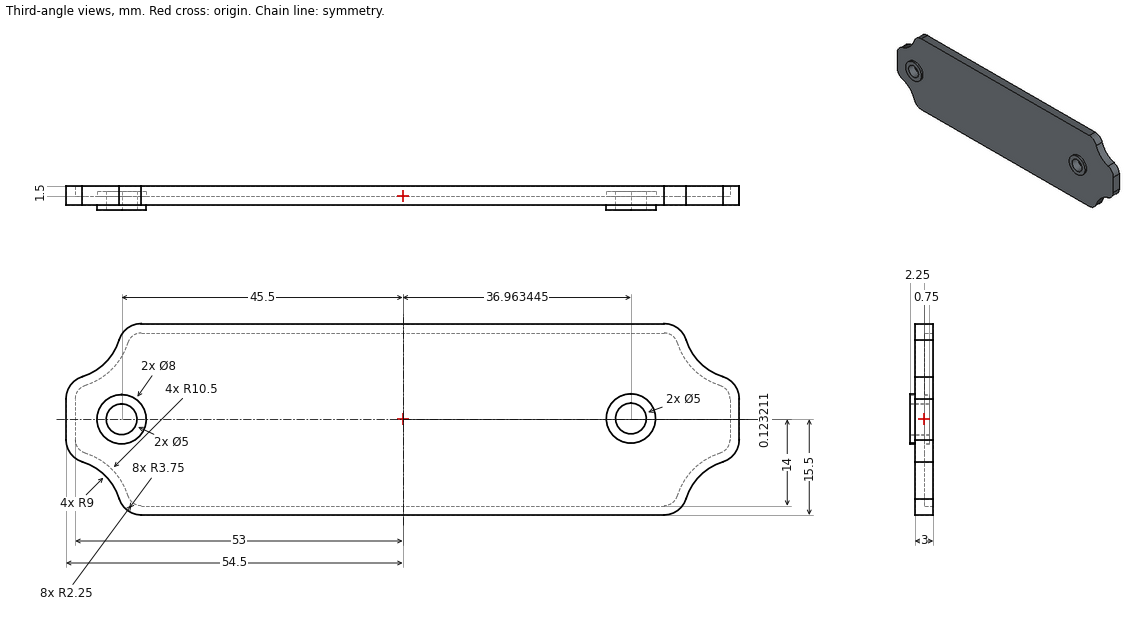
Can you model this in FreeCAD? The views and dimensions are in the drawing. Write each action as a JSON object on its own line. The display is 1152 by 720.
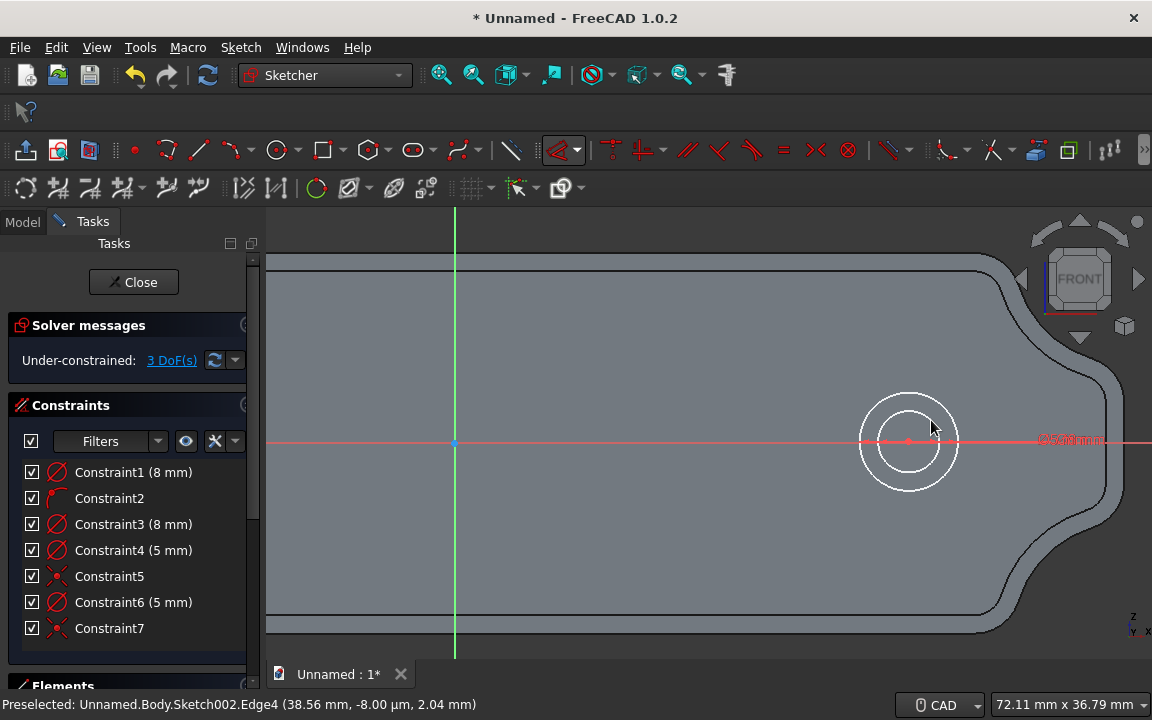
{"action": "scroll", "coordinate": [835, 425], "scroll_direction": "down", "scroll_amount": 4}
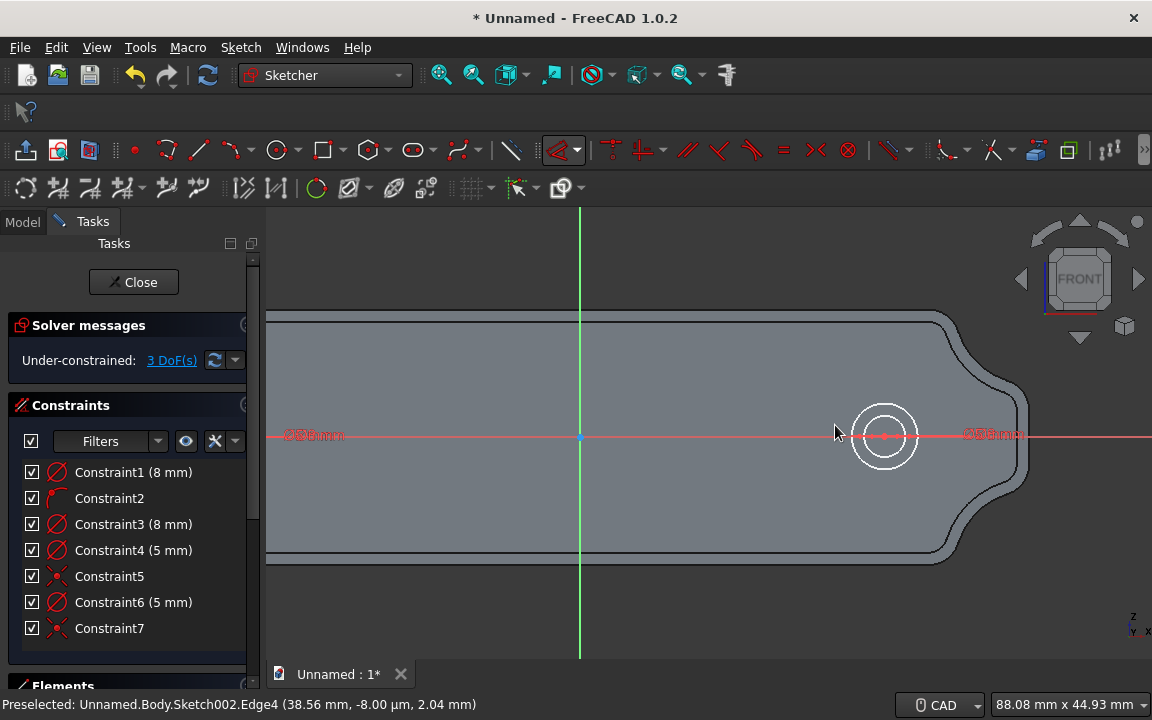
{"action": "left_click", "coordinate": [413, 433]}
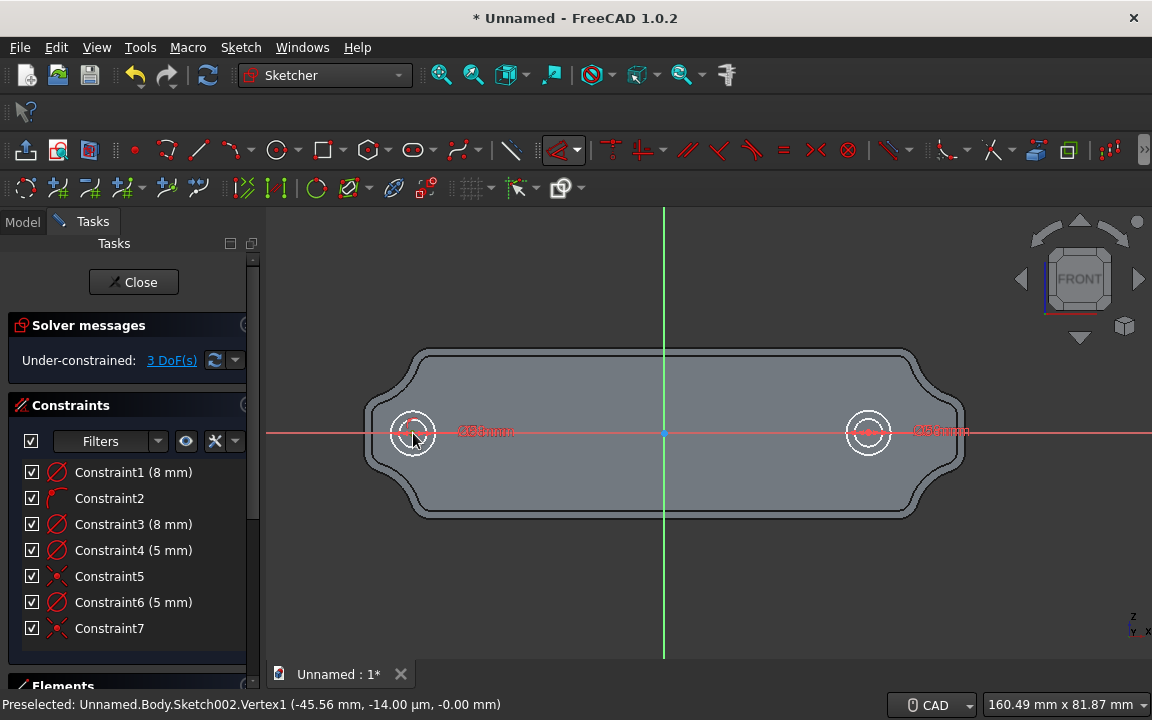
{"action": "key", "text": "l"}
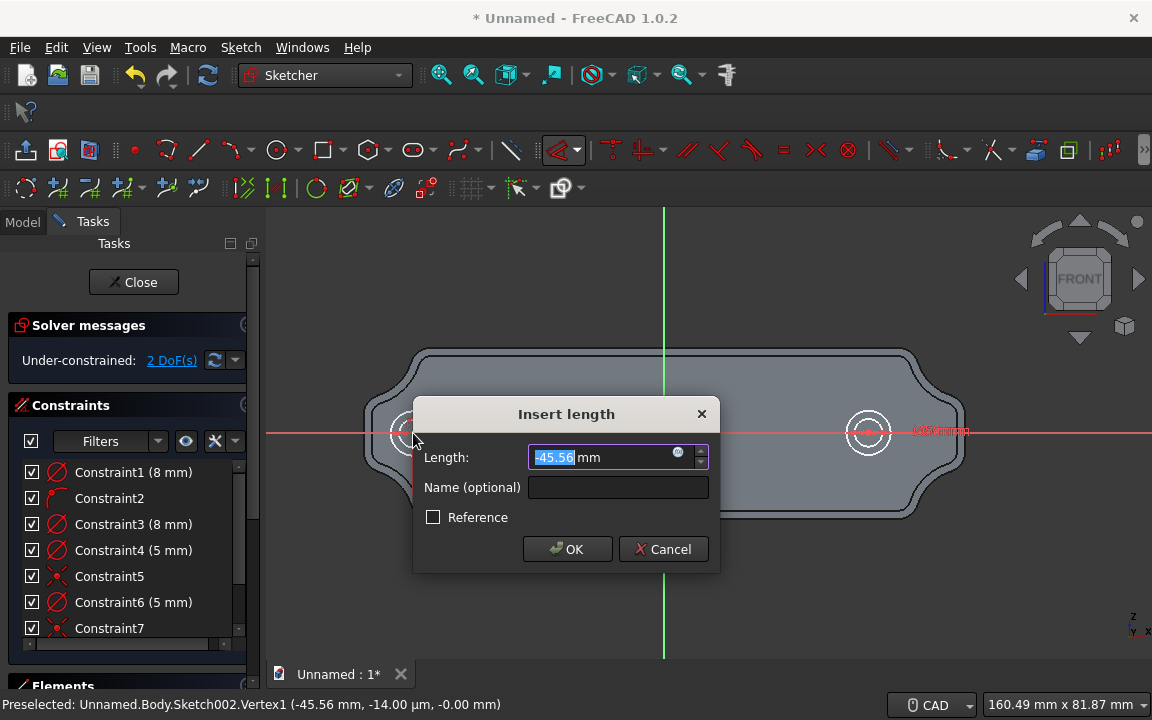
{"action": "type", "text": "-45.5"}
{"action": "key", "text": "Return"}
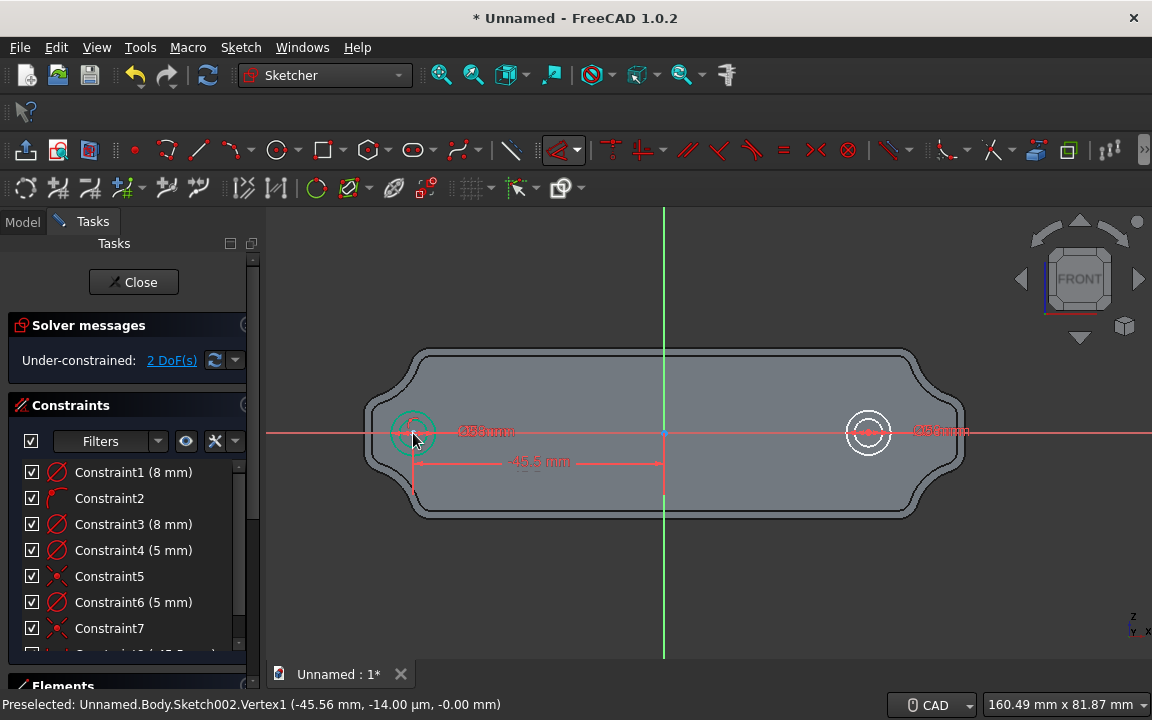
{"action": "scroll", "coordinate": [869, 433], "scroll_direction": "up", "scroll_amount": 21}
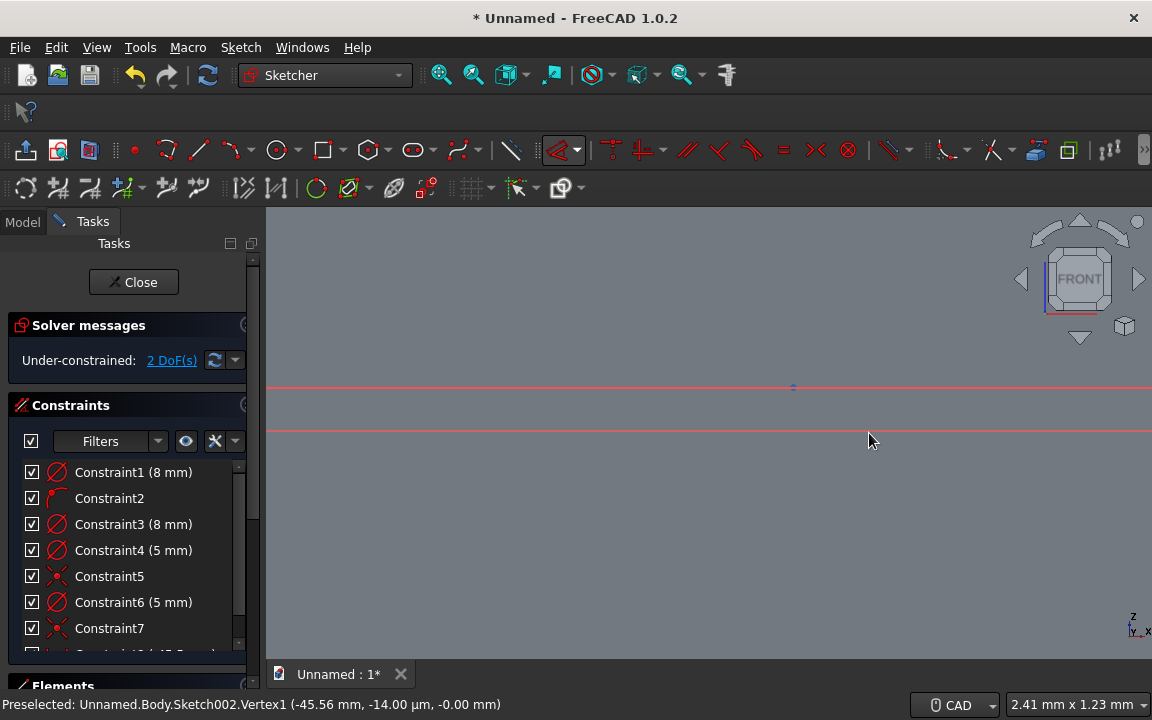
{"action": "left_click", "coordinate": [793, 388]}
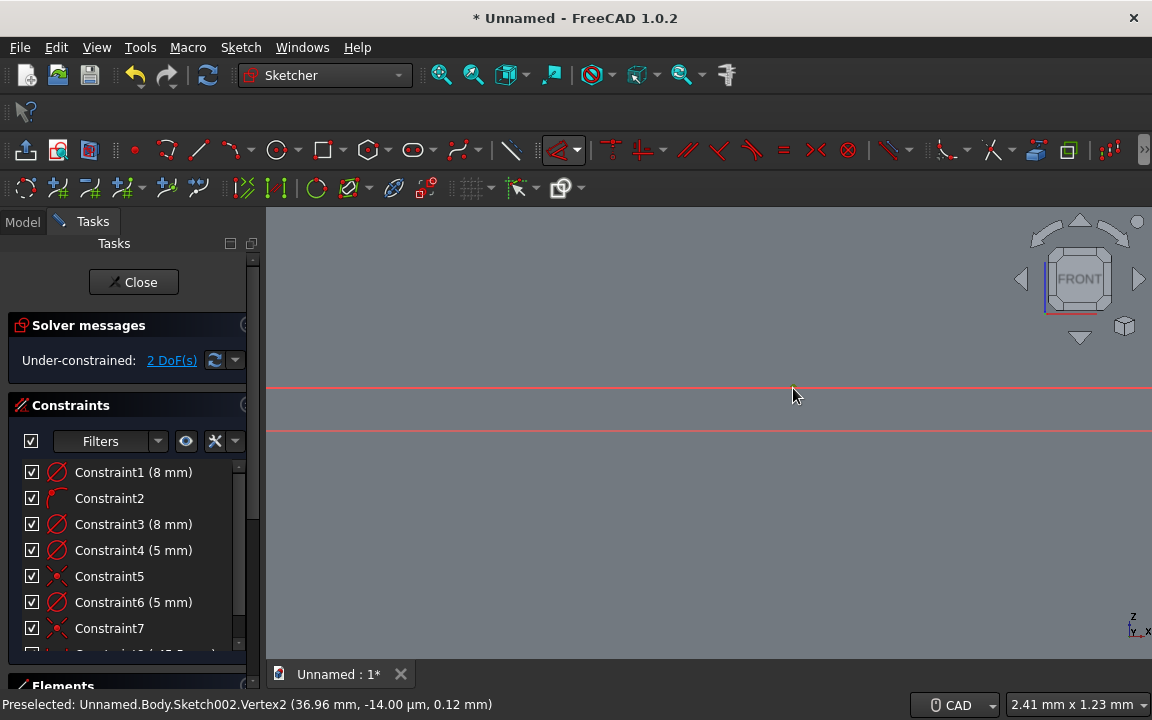
{"action": "left_click", "coordinate": [580, 150]}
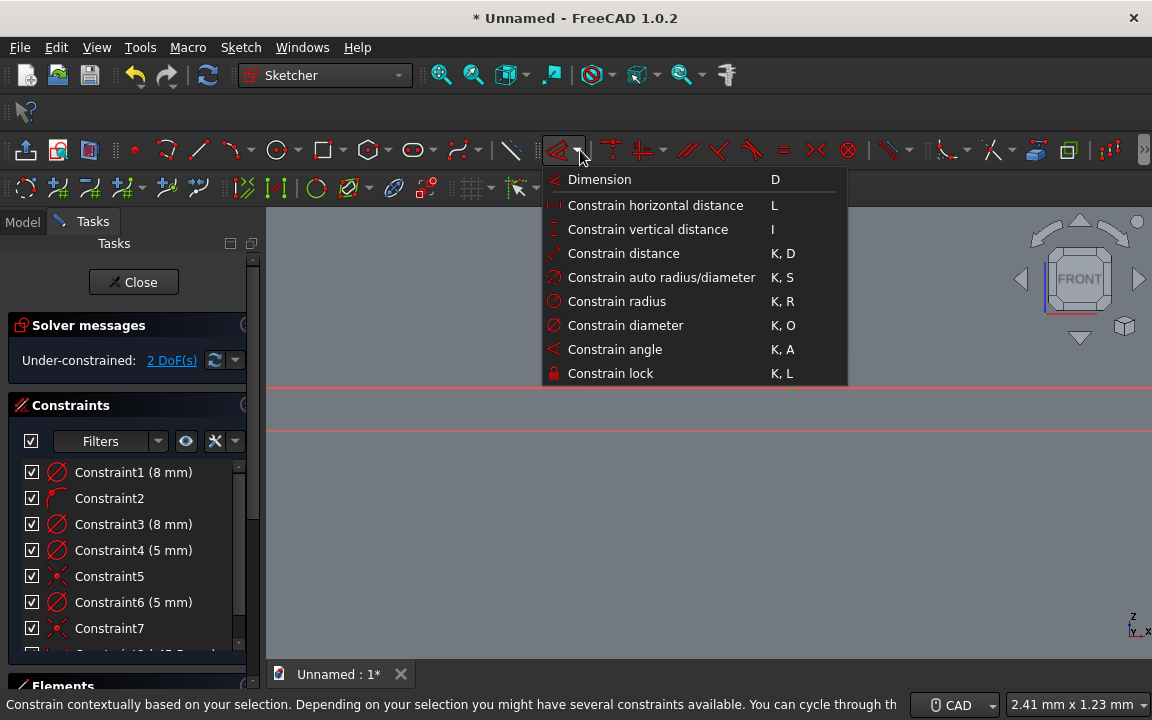
{"action": "left_click", "coordinate": [695, 229]}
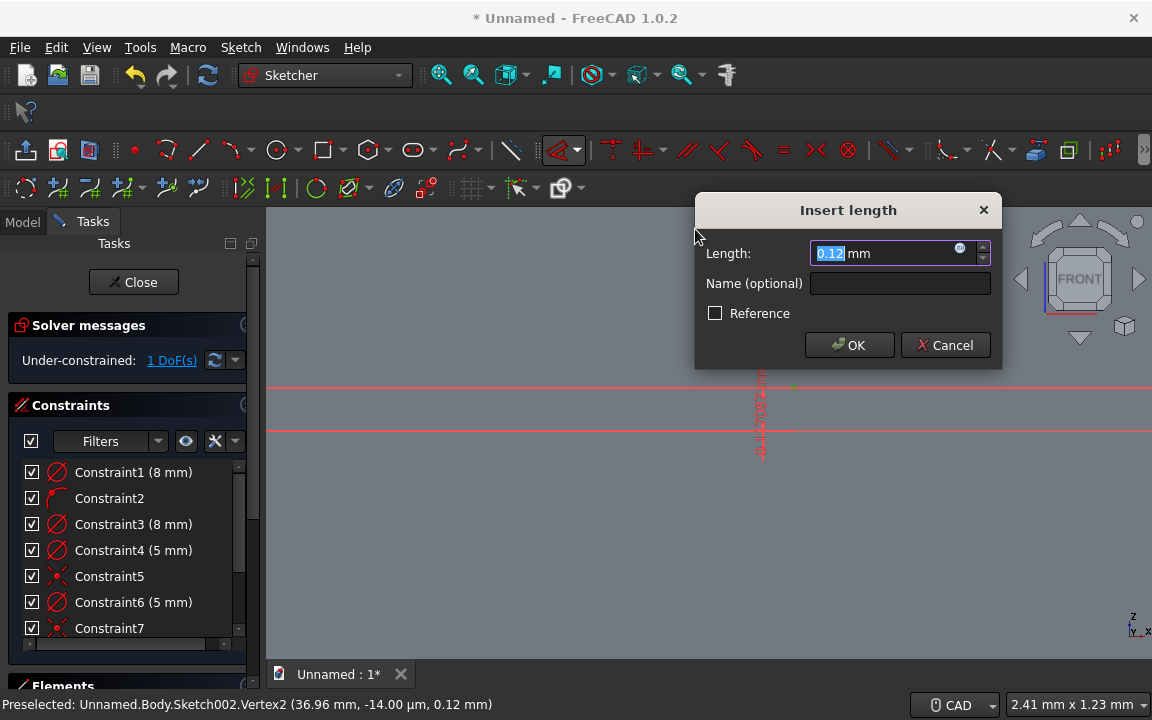
{"action": "type", "text": "0.123211"}
{"action": "key", "text": "Return"}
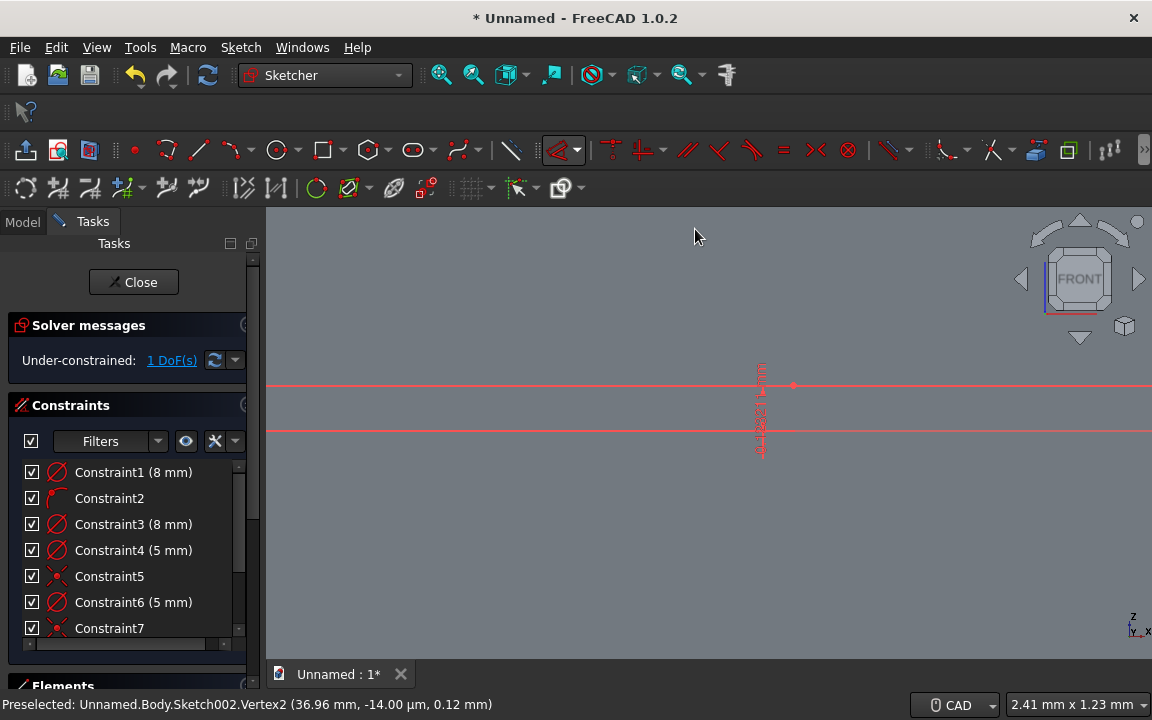
{"action": "scroll", "coordinate": [640, 433], "scroll_direction": "down", "scroll_amount": 15}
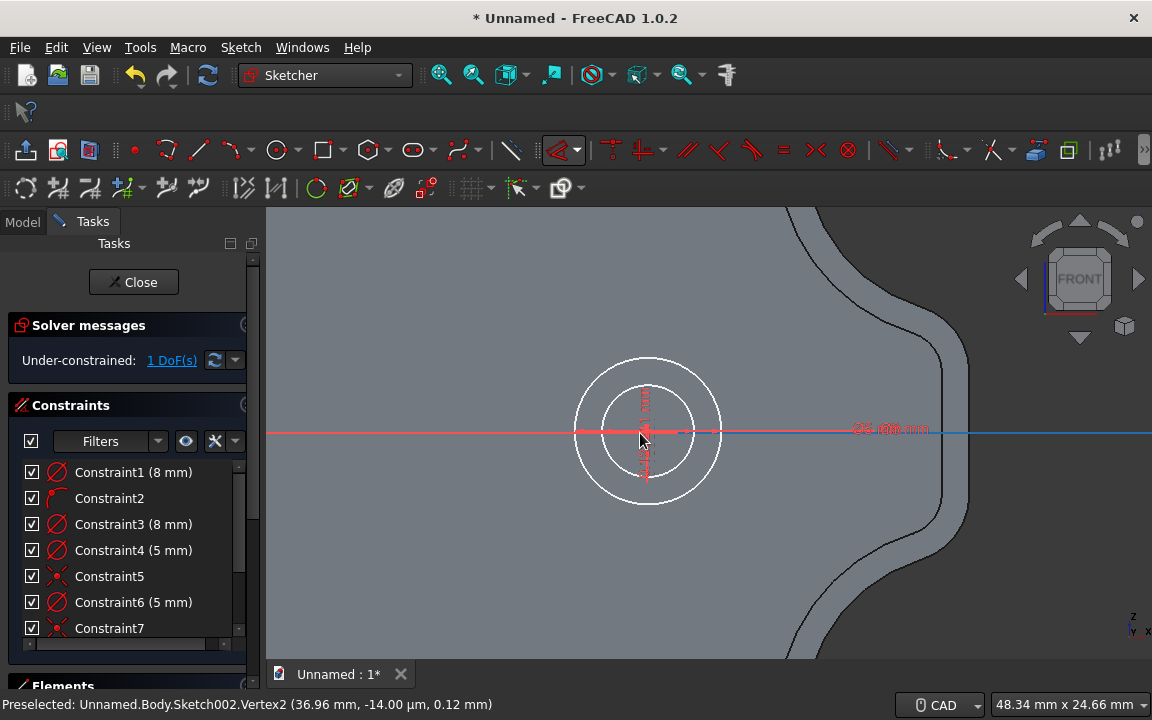
{"action": "scroll", "coordinate": [963, 433], "scroll_direction": "down", "scroll_amount": 6}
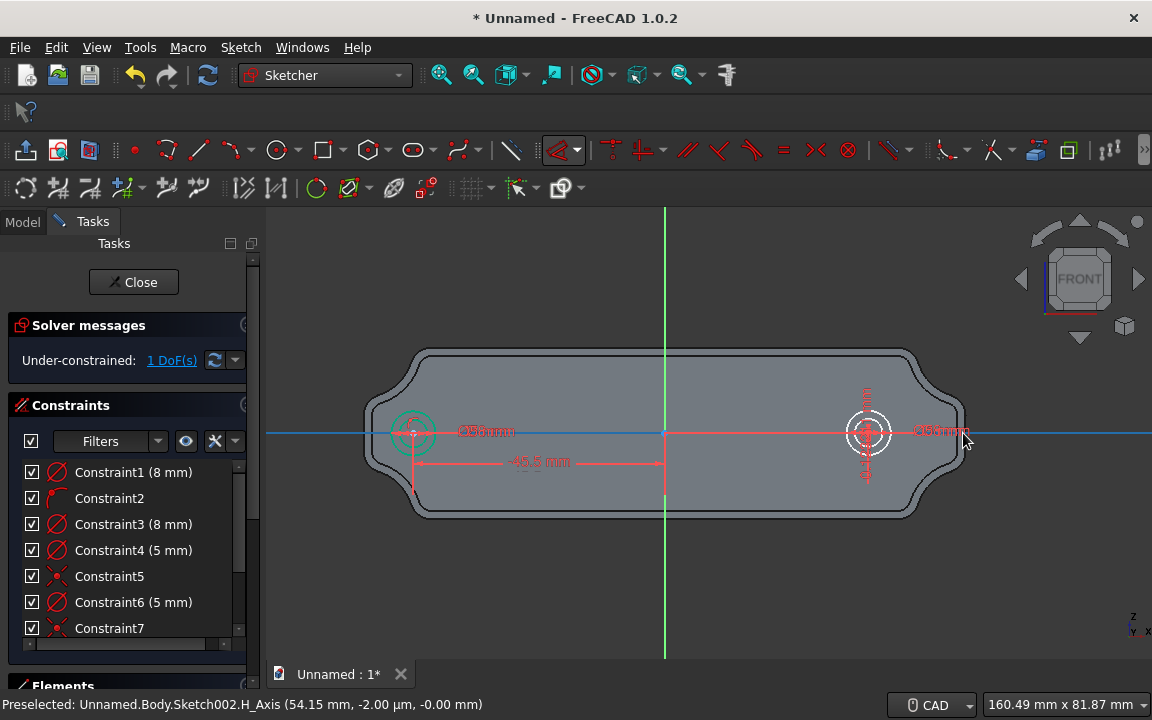
{"action": "left_click", "coordinate": [869, 433]}